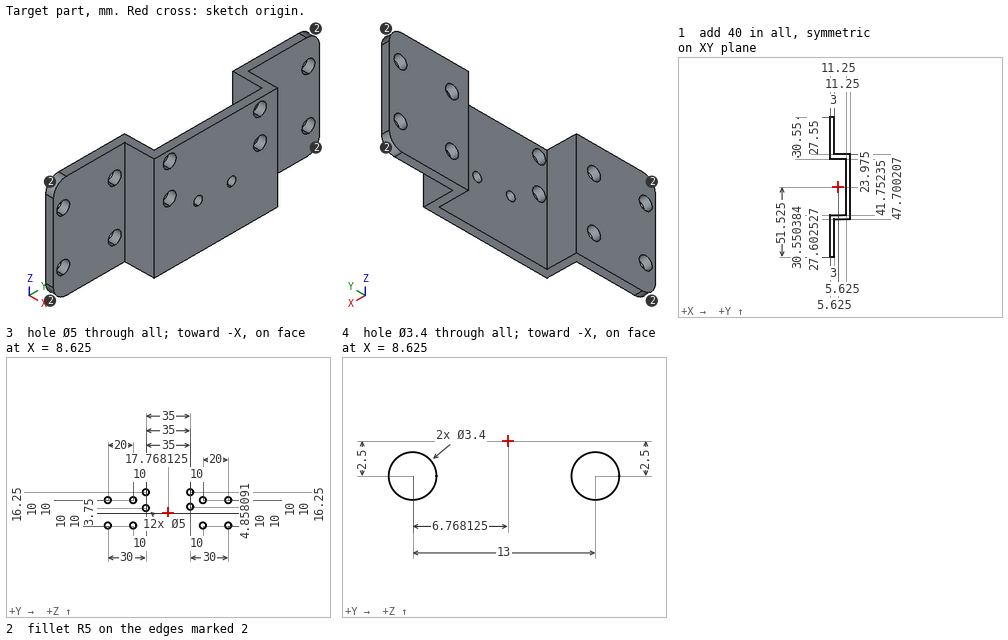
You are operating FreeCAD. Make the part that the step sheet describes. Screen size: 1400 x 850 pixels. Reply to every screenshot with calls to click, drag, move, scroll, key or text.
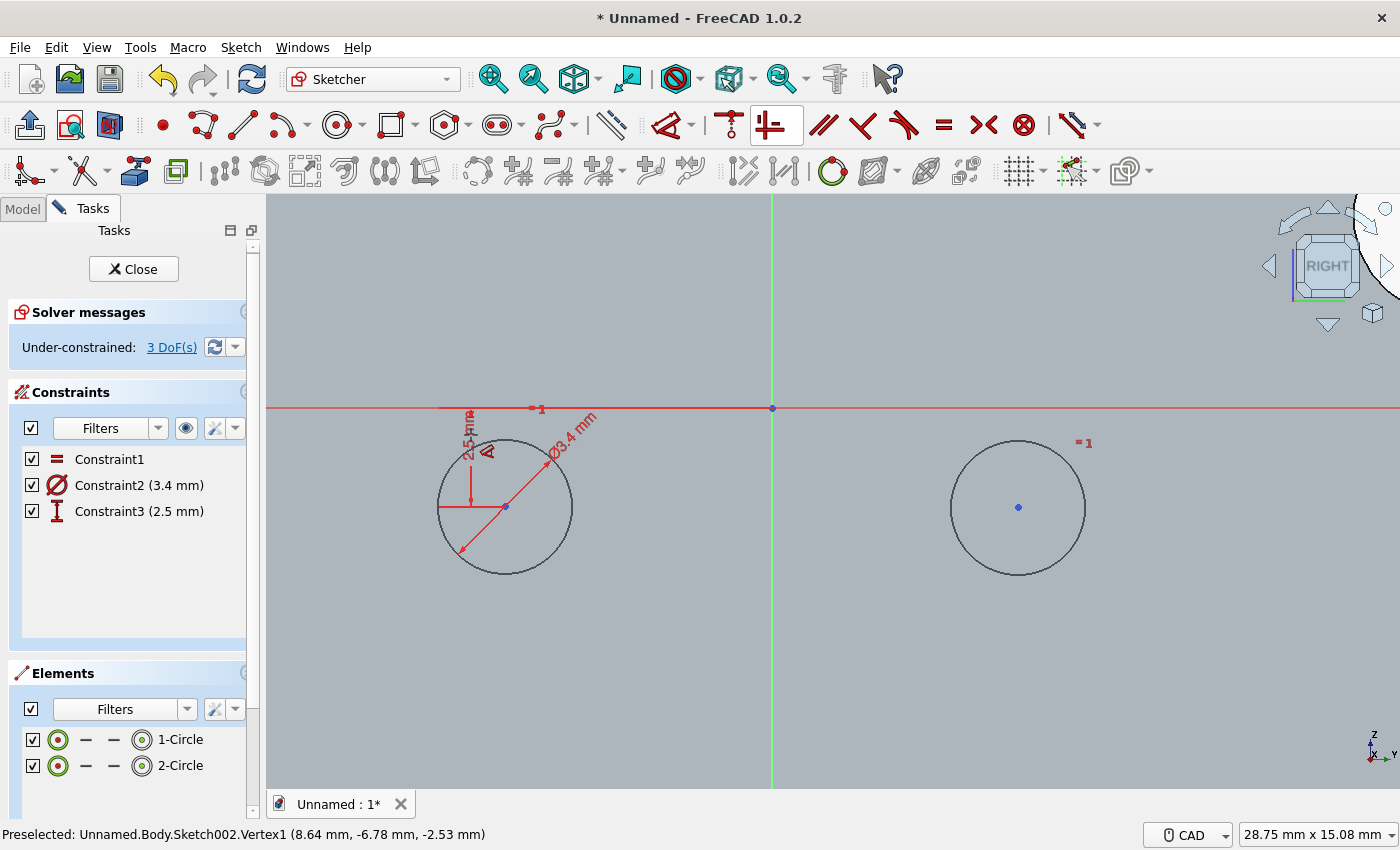
click(1018, 508)
click(1052, 435)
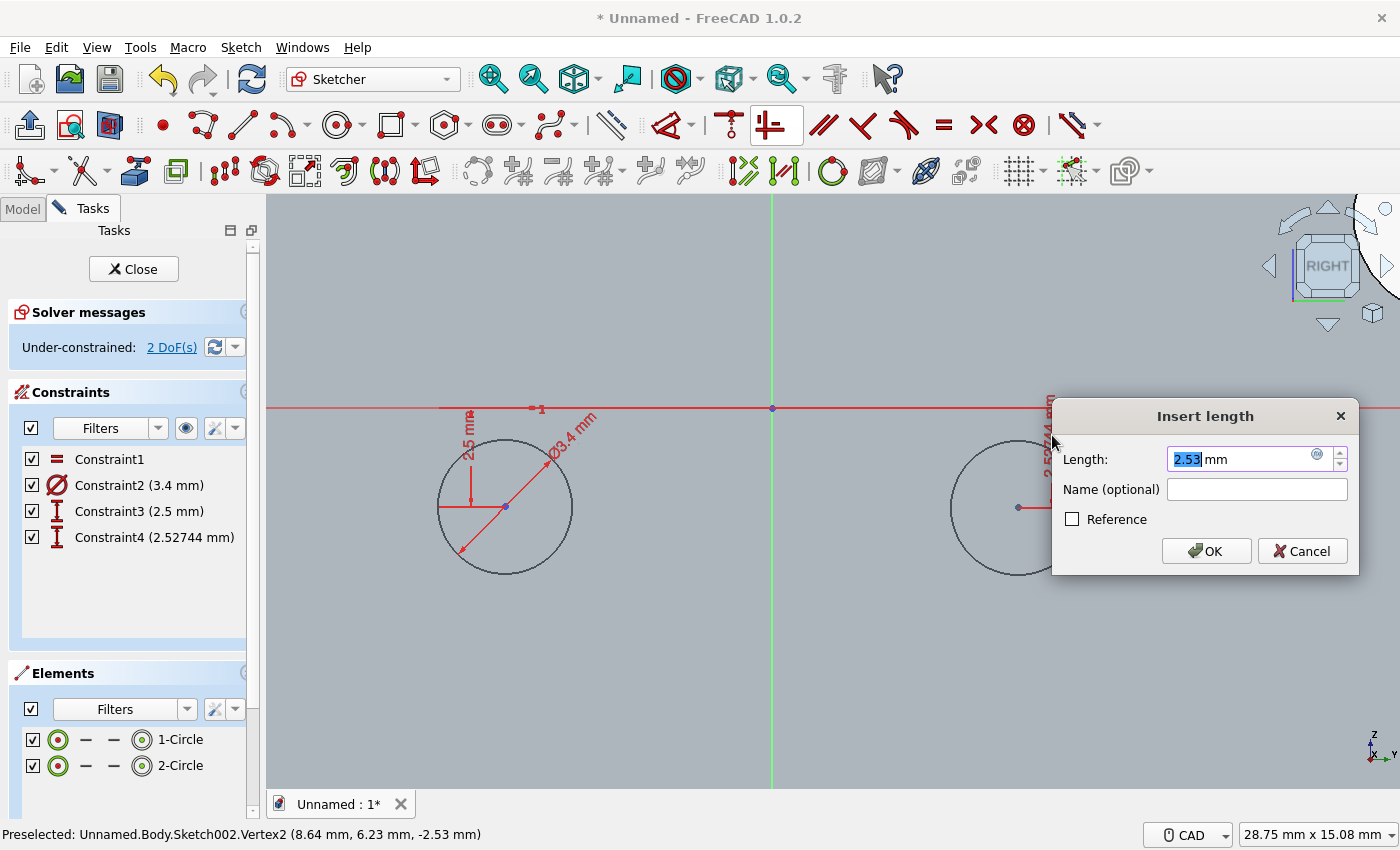
text(2.5)
key(Return)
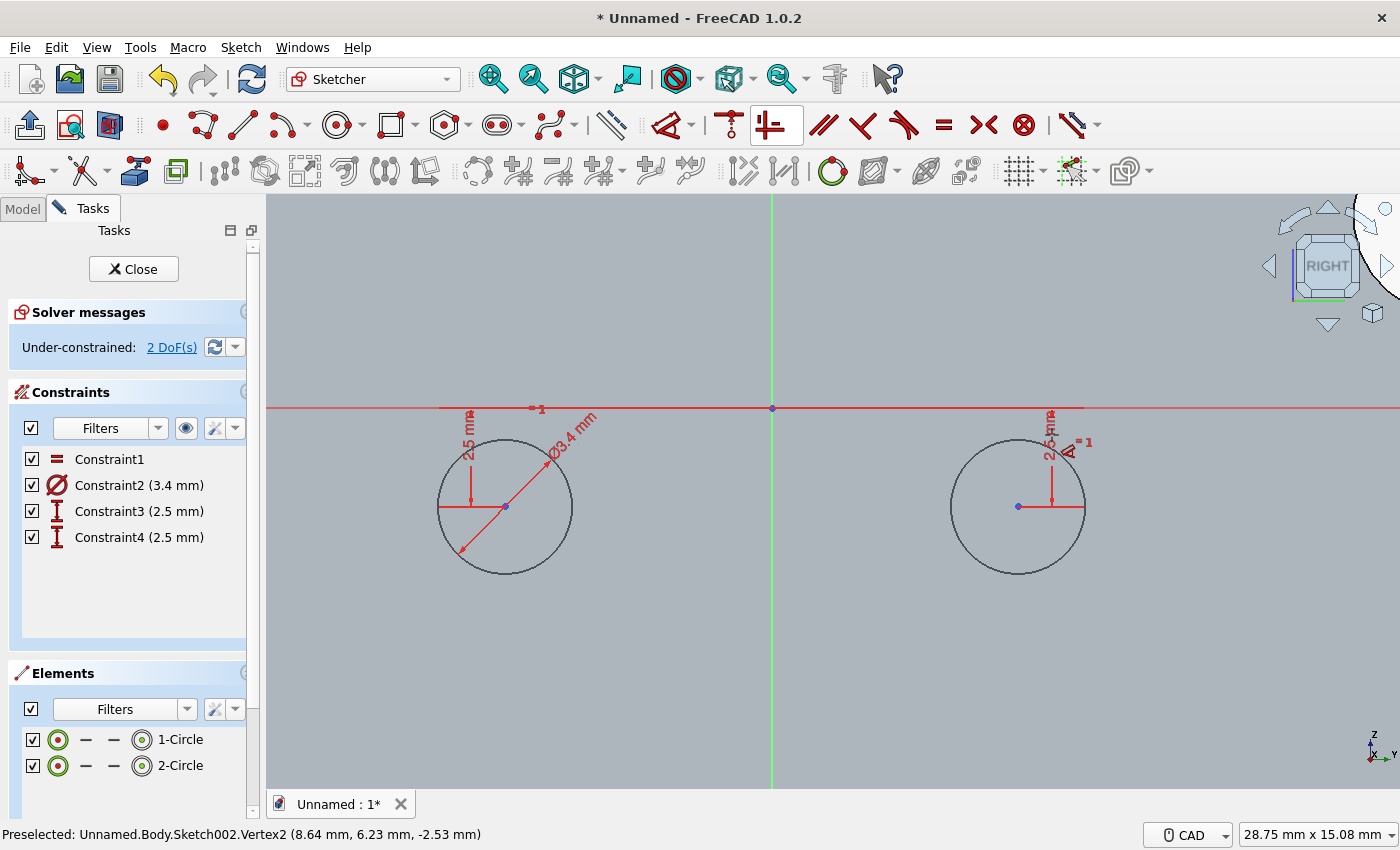
click(505, 507)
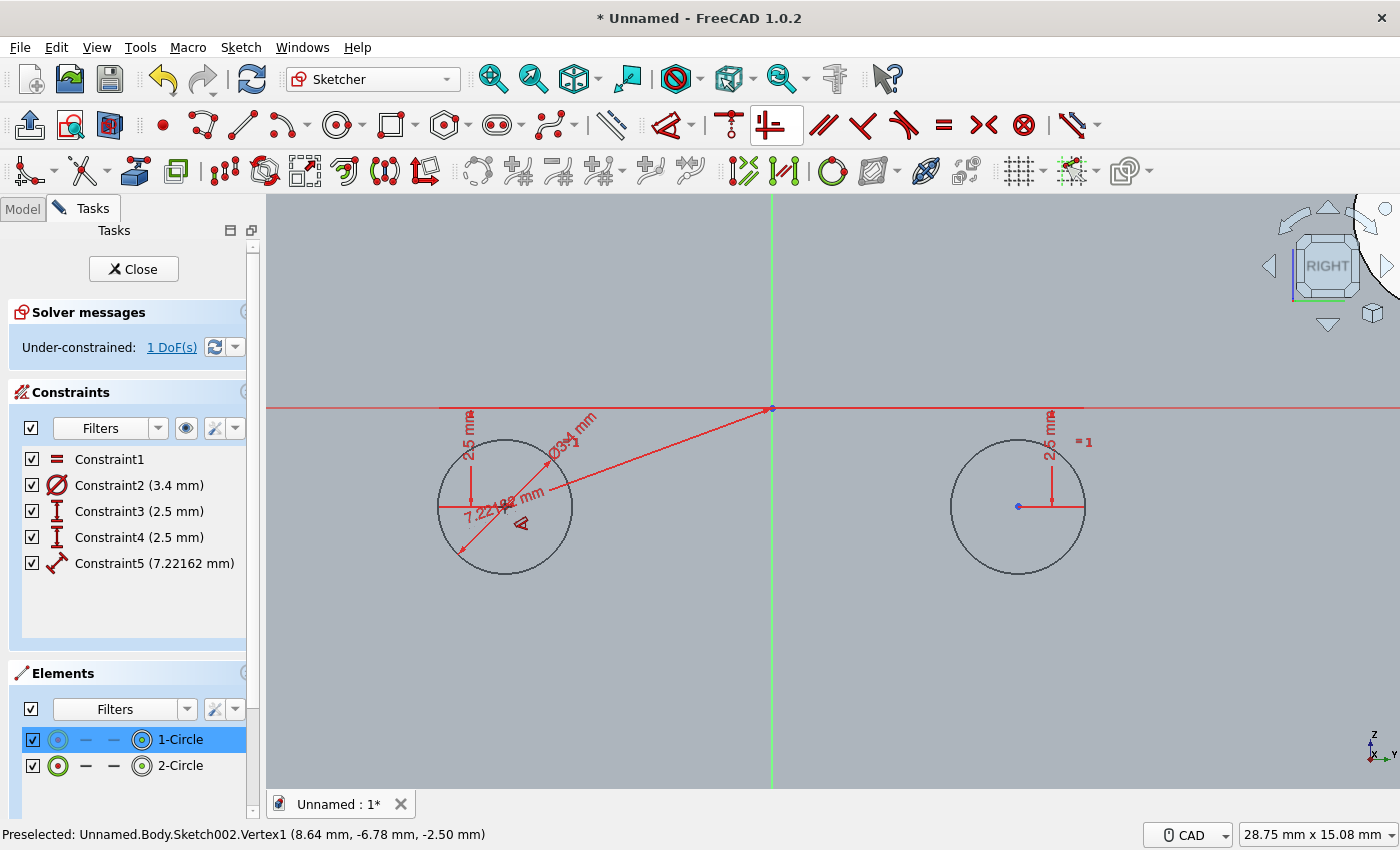
click(1018, 507)
click(644, 541)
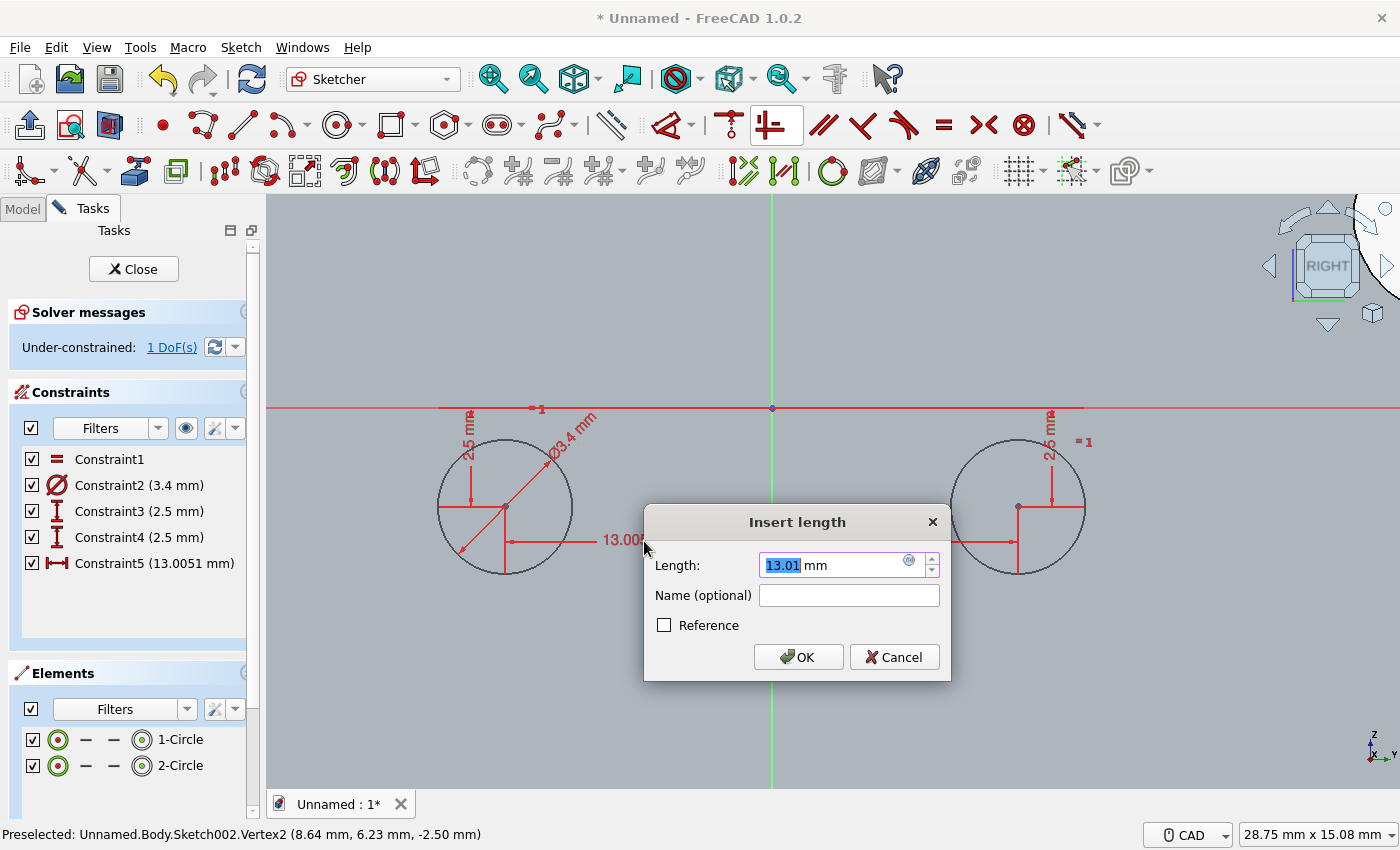
text(13)
key(Return)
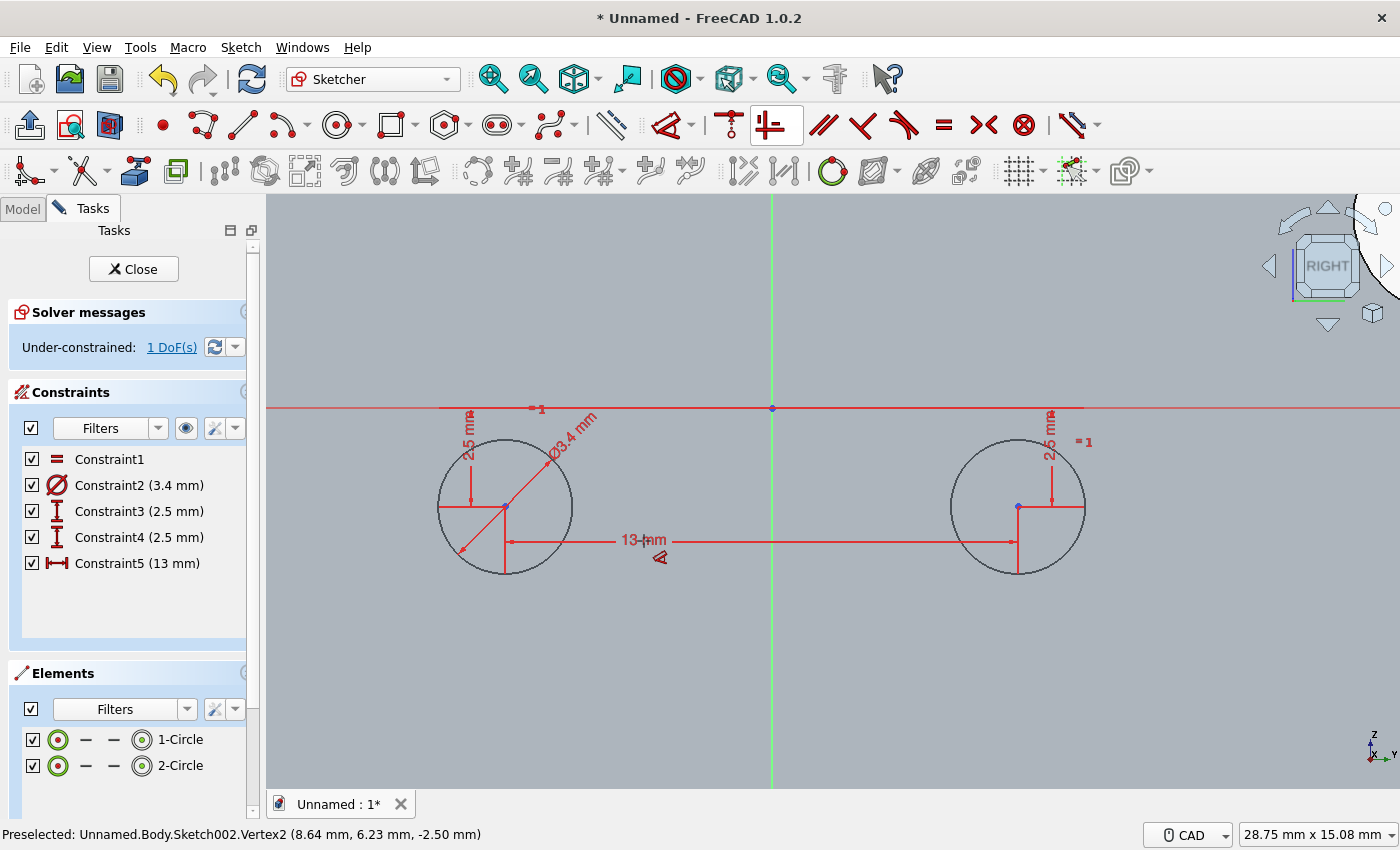
click(505, 507)
click(639, 374)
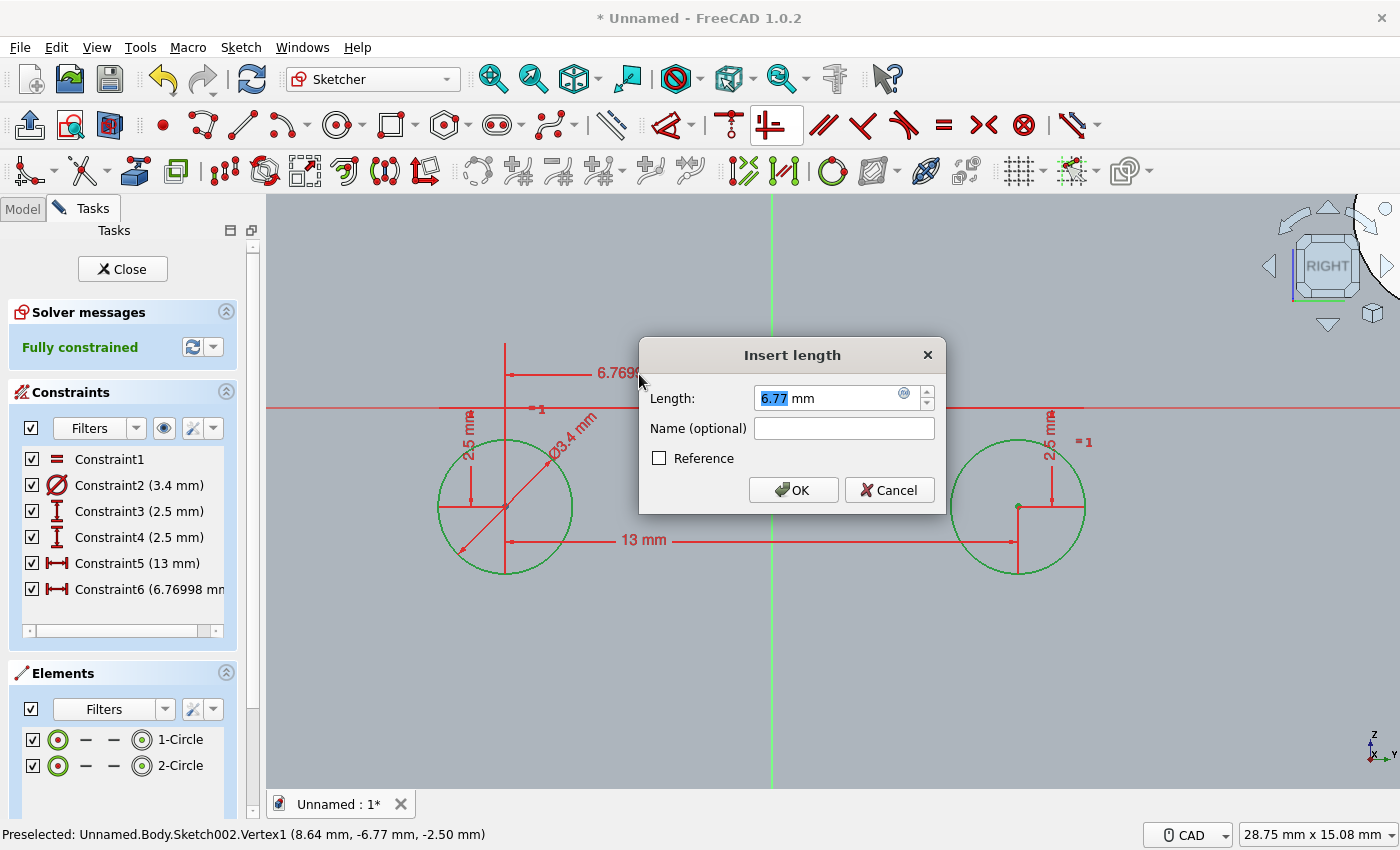
text(6.768125)
key(Return)
key(Escape)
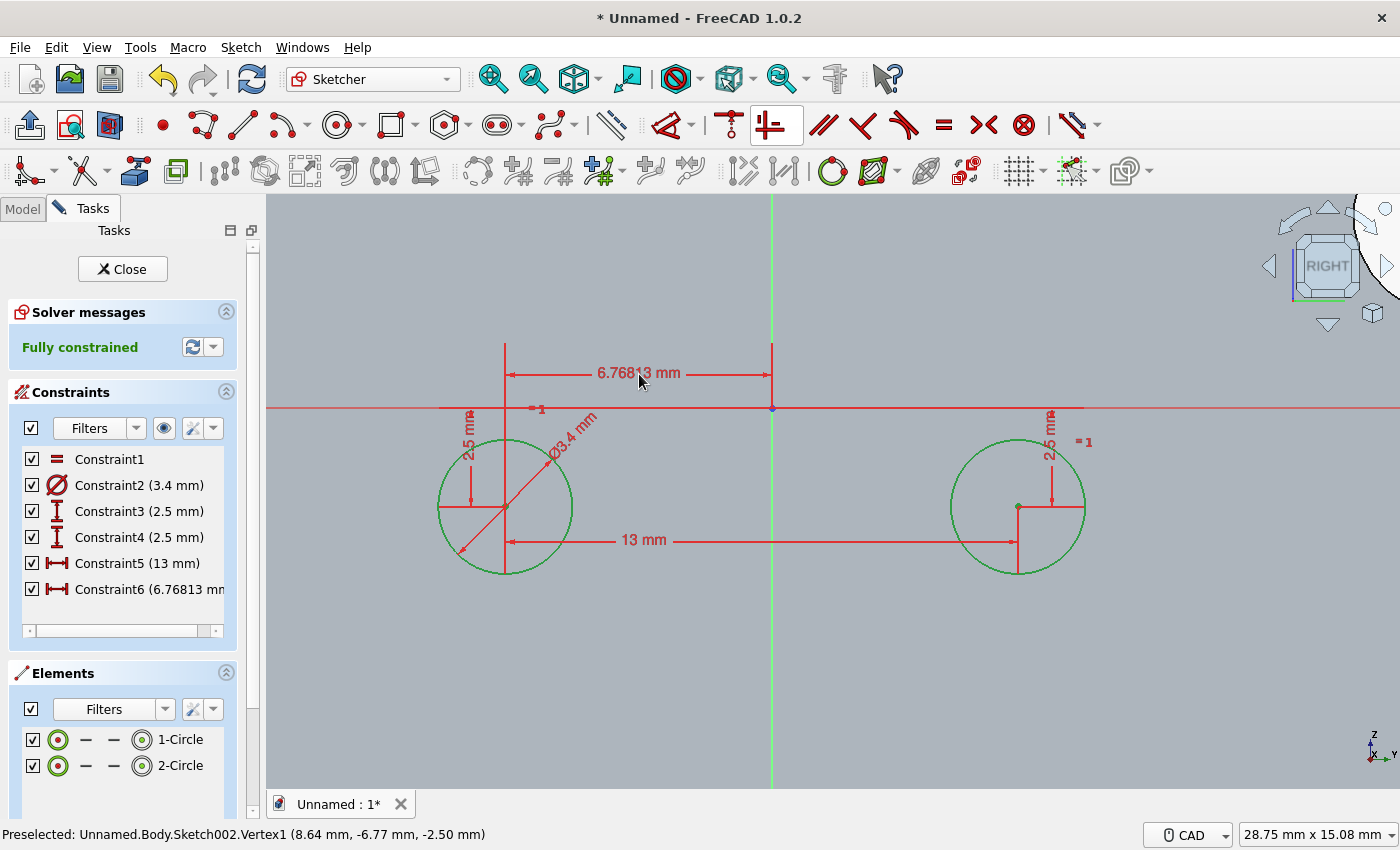
click(123, 269)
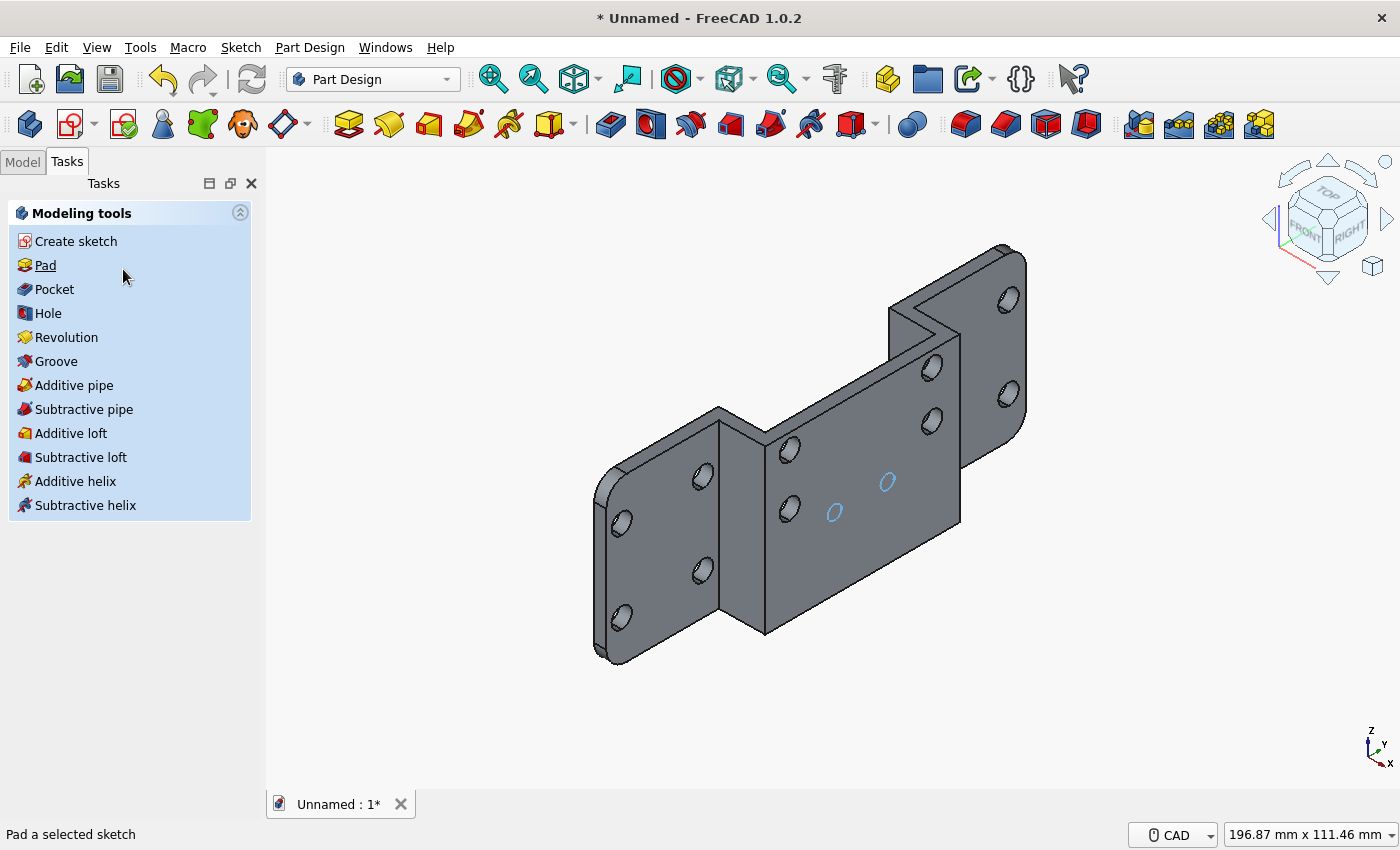
click(652, 124)